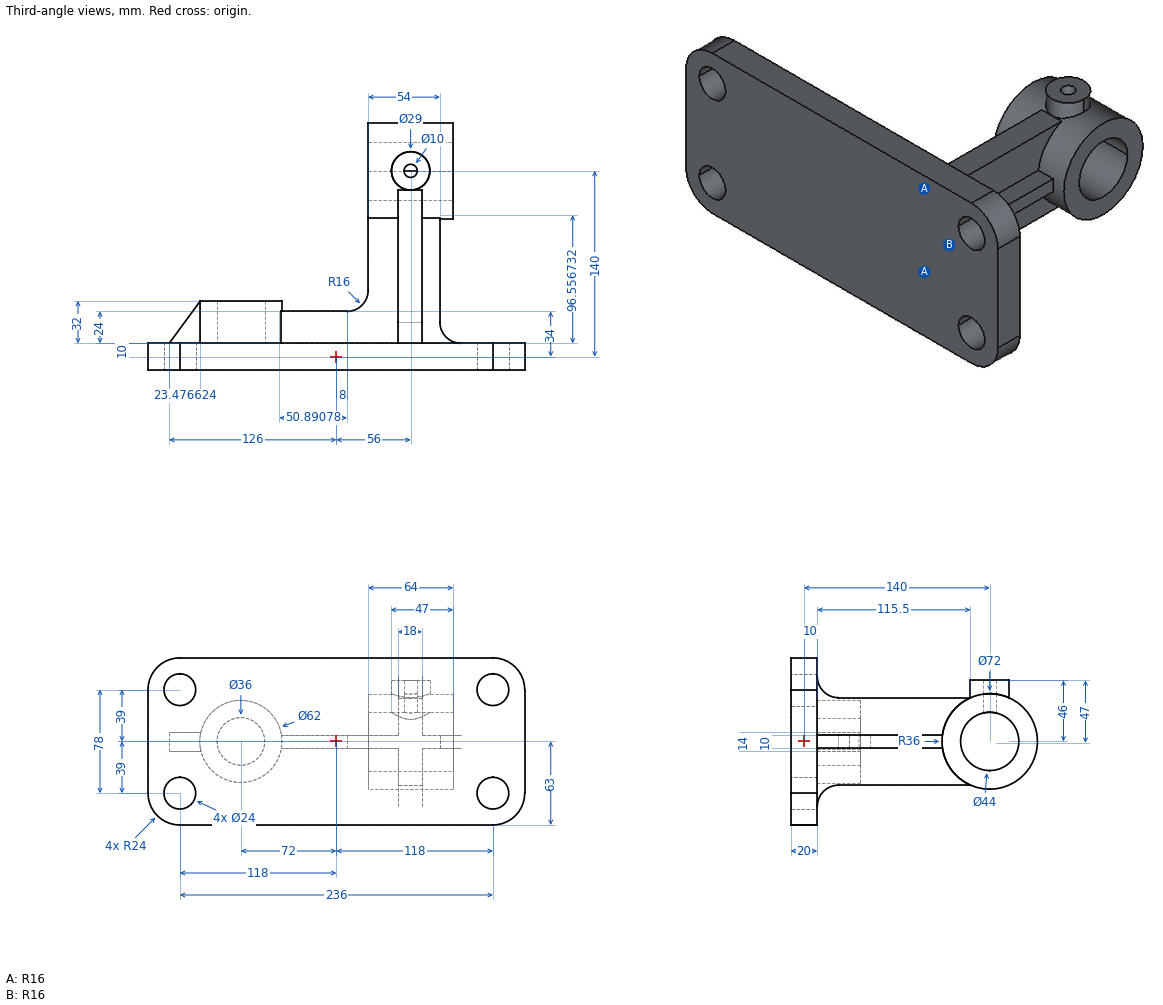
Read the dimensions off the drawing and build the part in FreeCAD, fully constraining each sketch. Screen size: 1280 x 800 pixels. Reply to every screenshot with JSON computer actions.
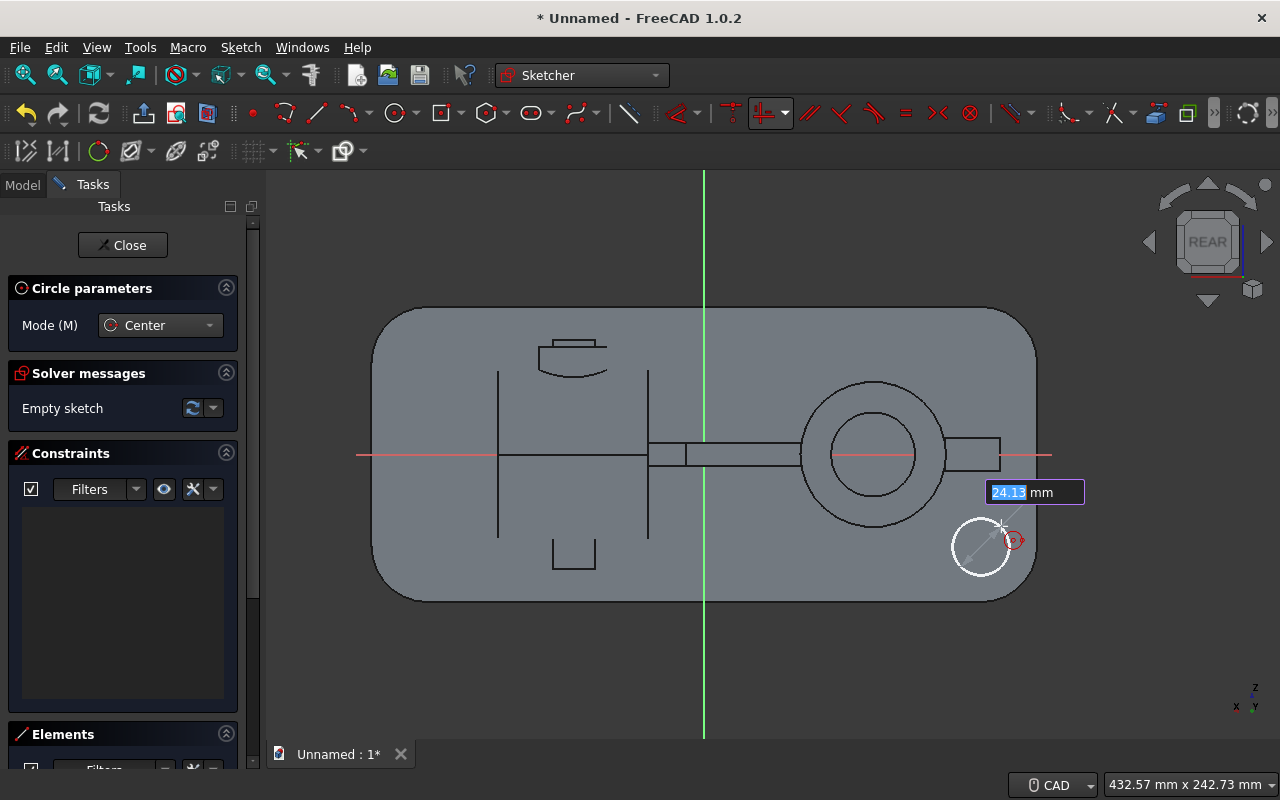
{"action": "type", "text": "24"}
{"action": "key", "text": "Return"}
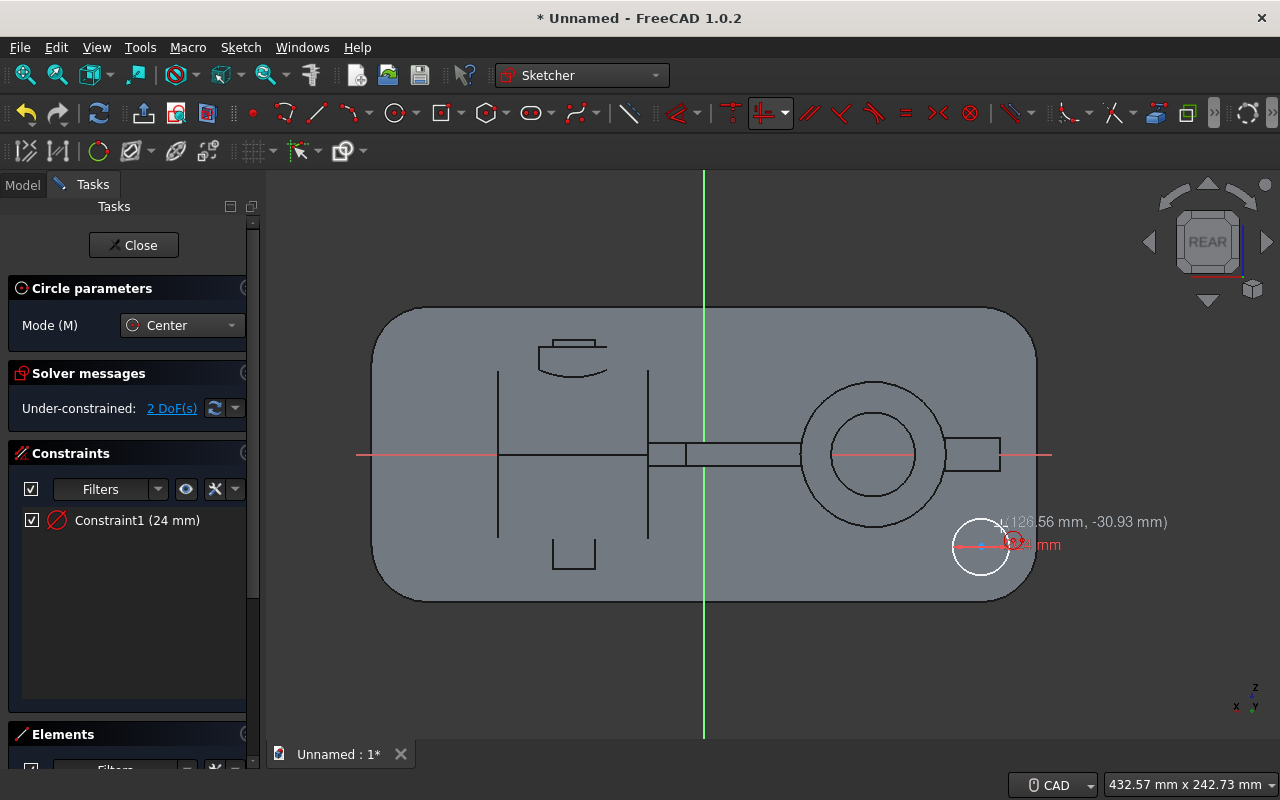
{"action": "left_click", "coordinate": [981, 363]}
{"action": "mouse_move", "coordinate": [1001, 343]}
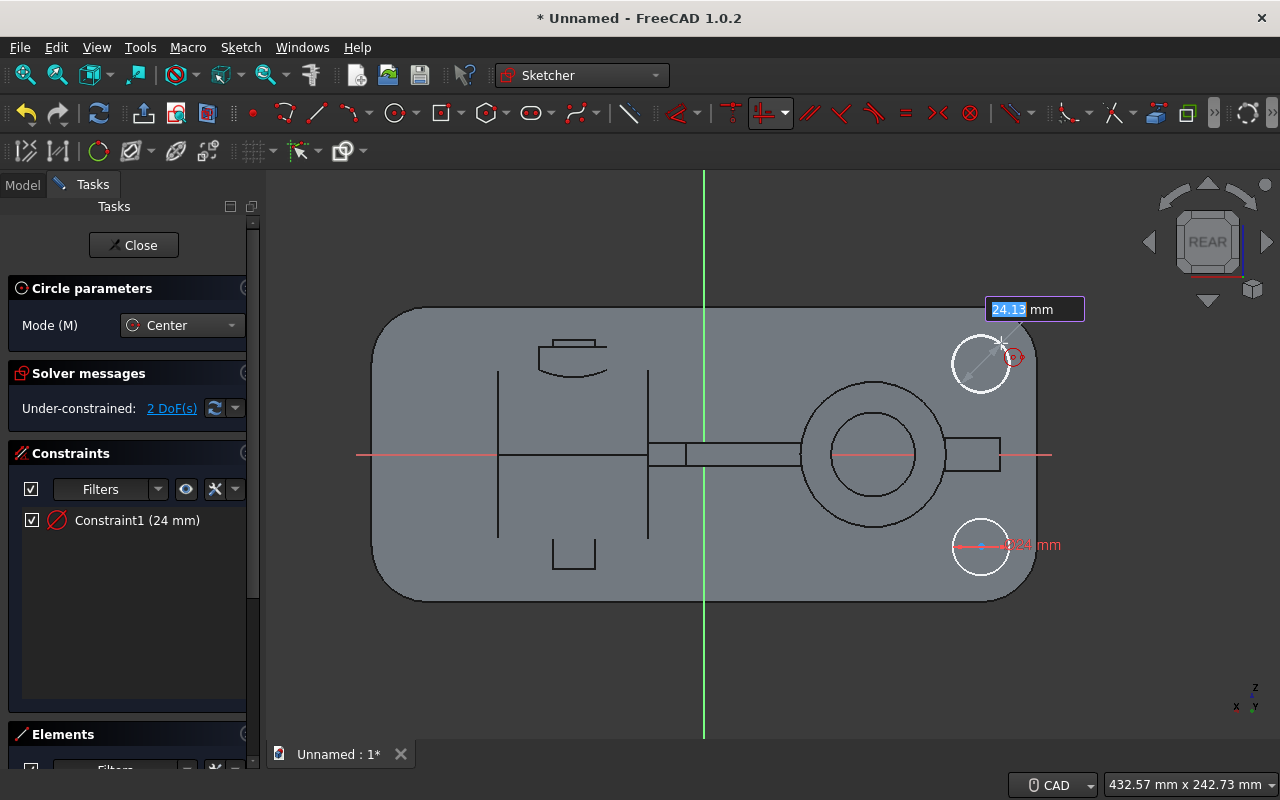
{"action": "type", "text": "24"}
{"action": "key", "text": "Return"}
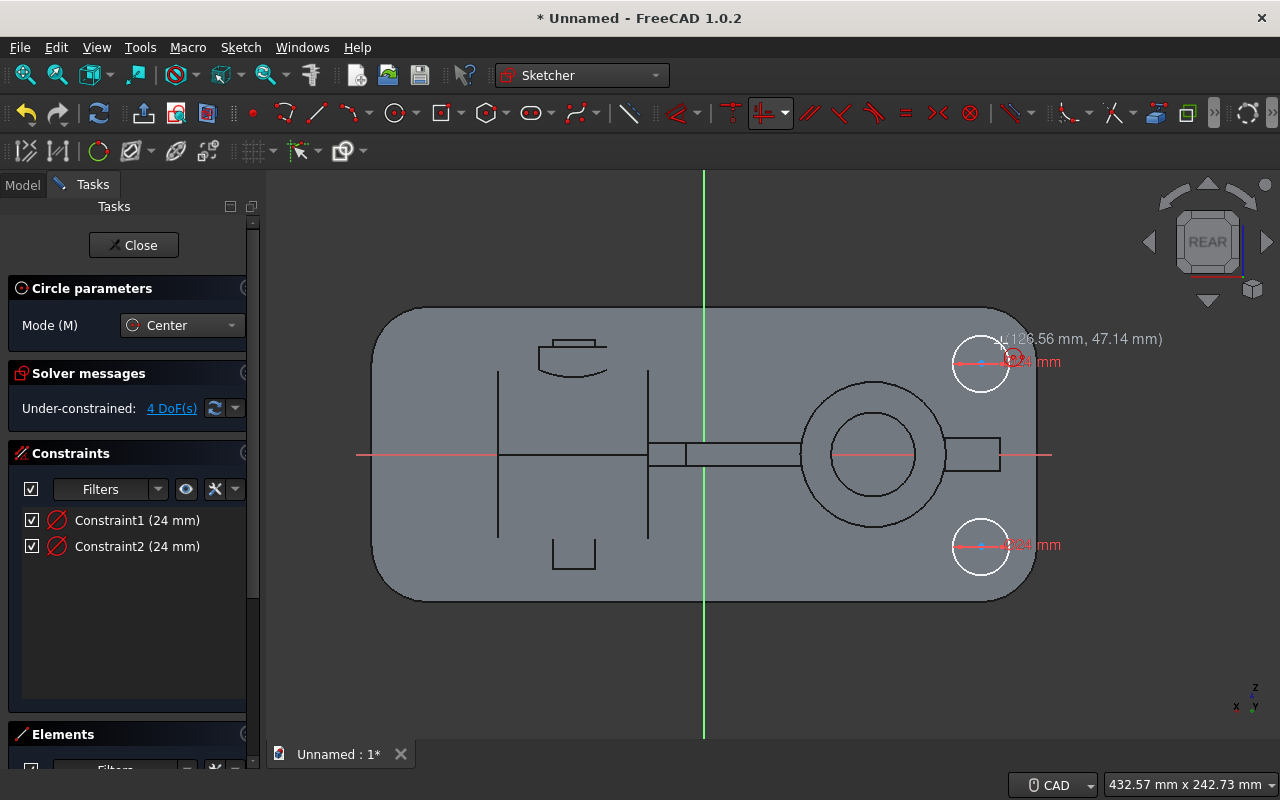
{"action": "left_click", "coordinate": [428, 363]}
{"action": "mouse_move", "coordinate": [448, 343]}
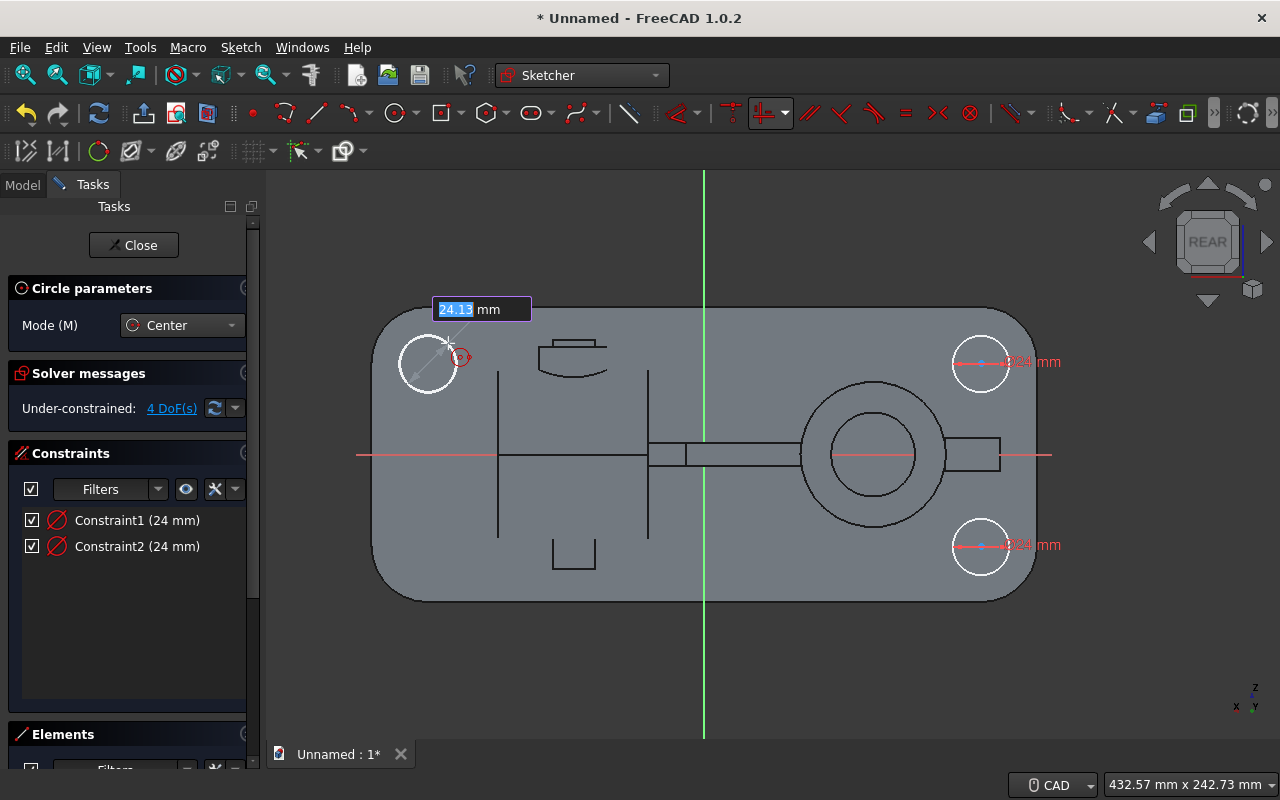
{"action": "type", "text": "24"}
{"action": "key", "text": "Return"}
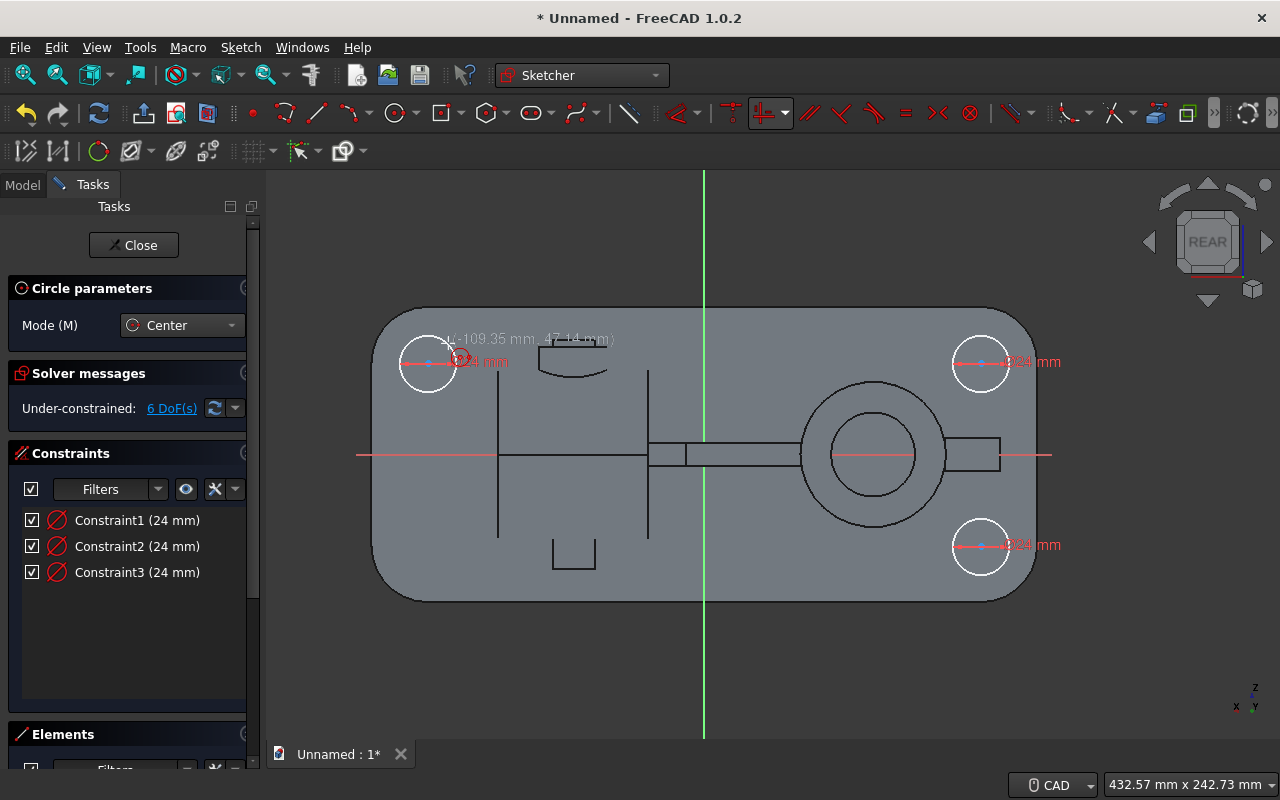
{"action": "left_click", "coordinate": [428, 546]}
{"action": "mouse_move", "coordinate": [448, 526]}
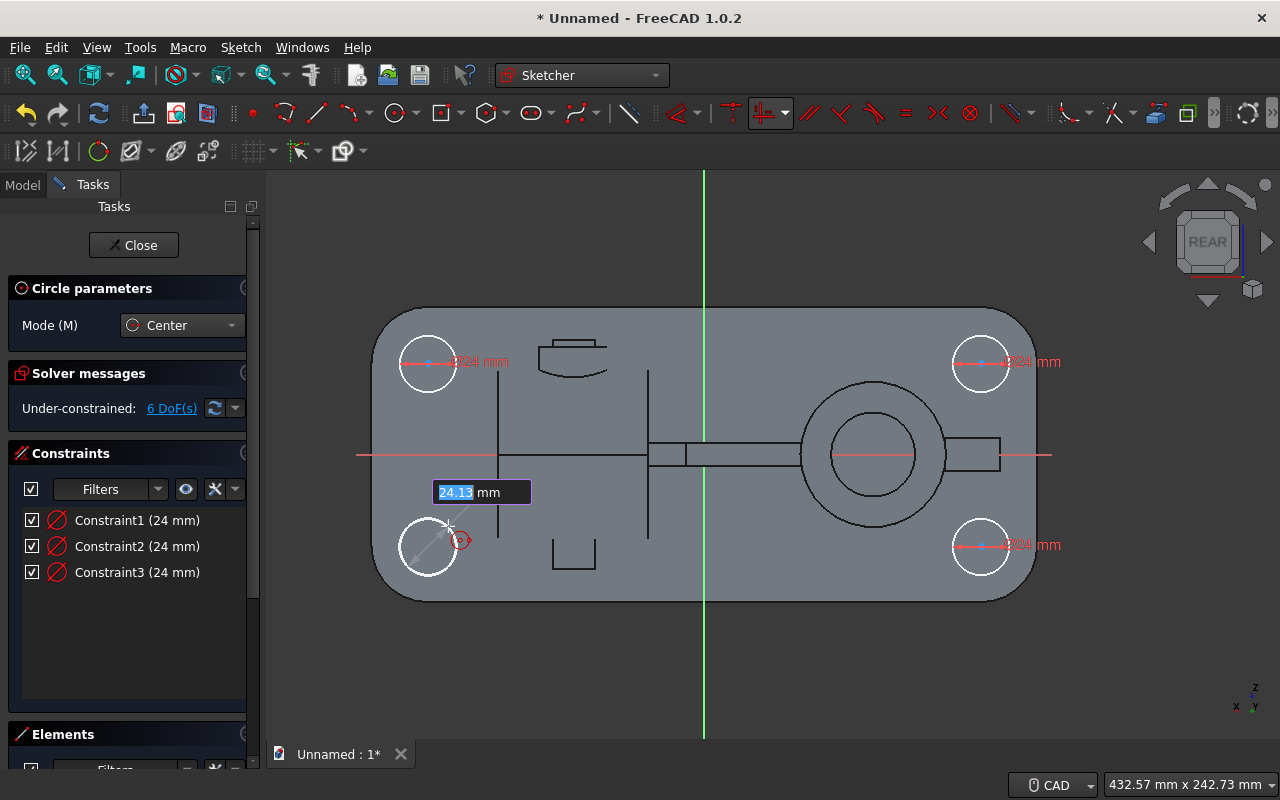
{"action": "type", "text": "24"}
{"action": "key", "text": "Return"}
{"action": "key", "text": "Escape"}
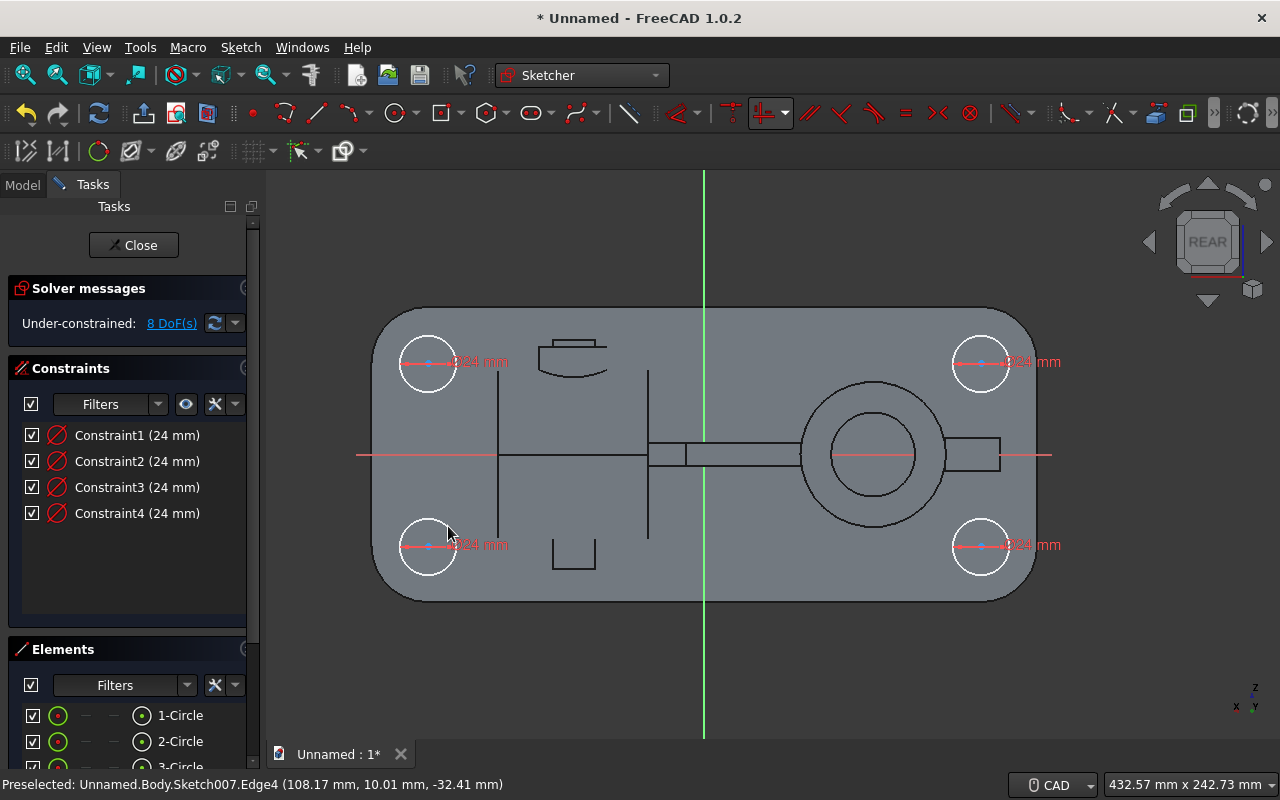
{"action": "left_click", "coordinate": [981, 547]}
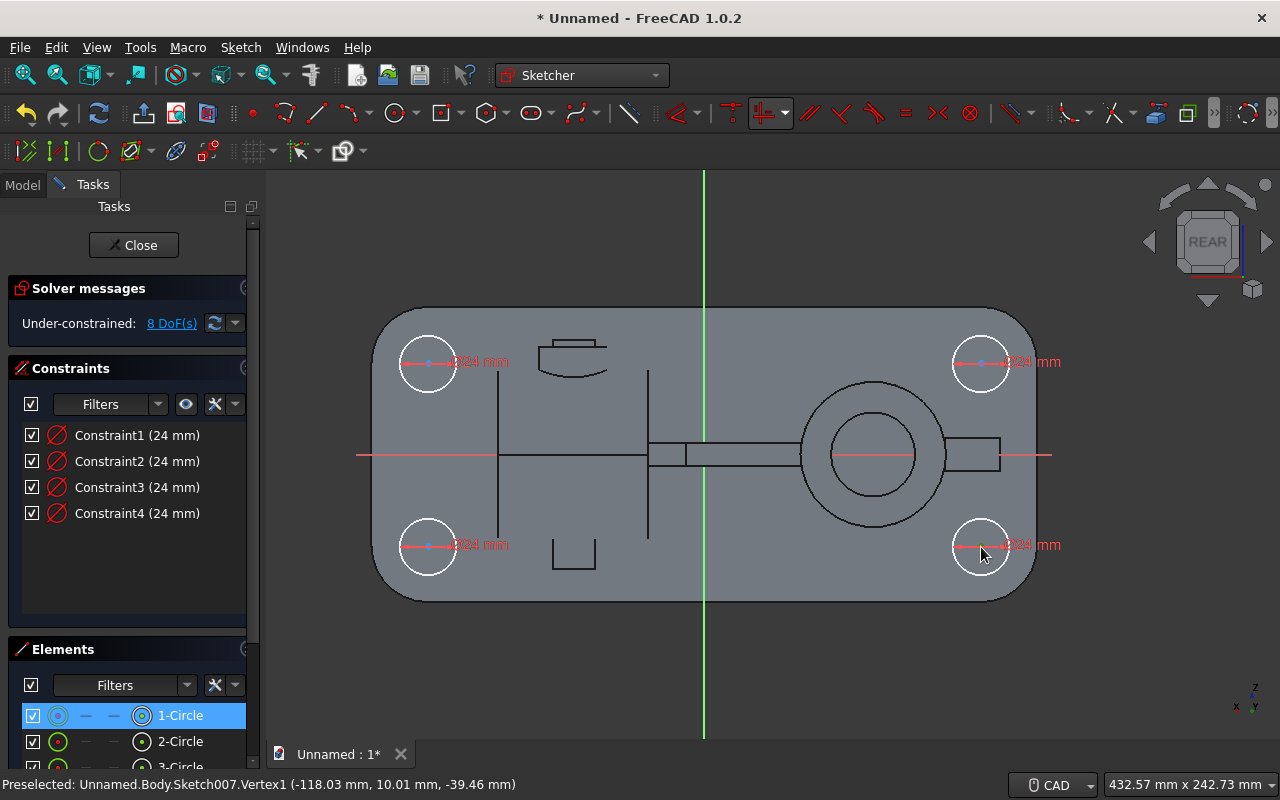
{"action": "left_click", "coordinate": [981, 364]}